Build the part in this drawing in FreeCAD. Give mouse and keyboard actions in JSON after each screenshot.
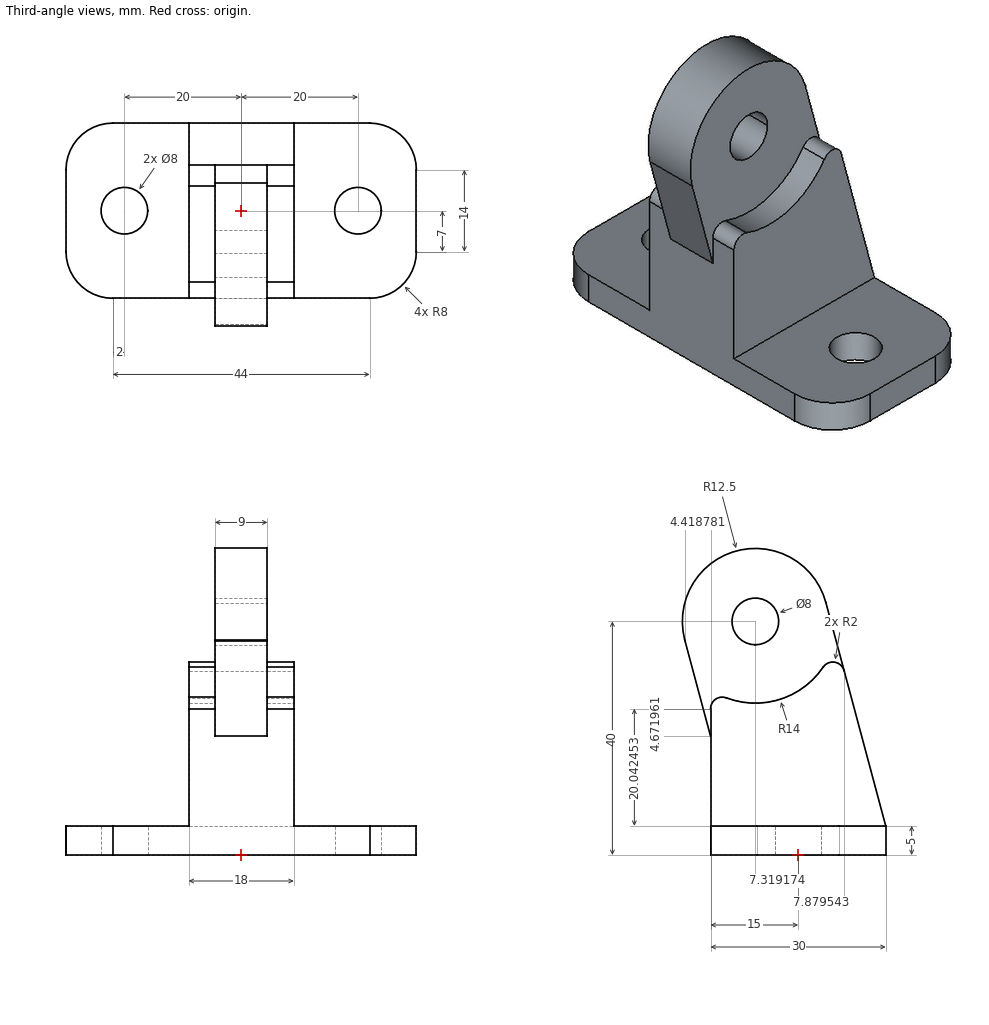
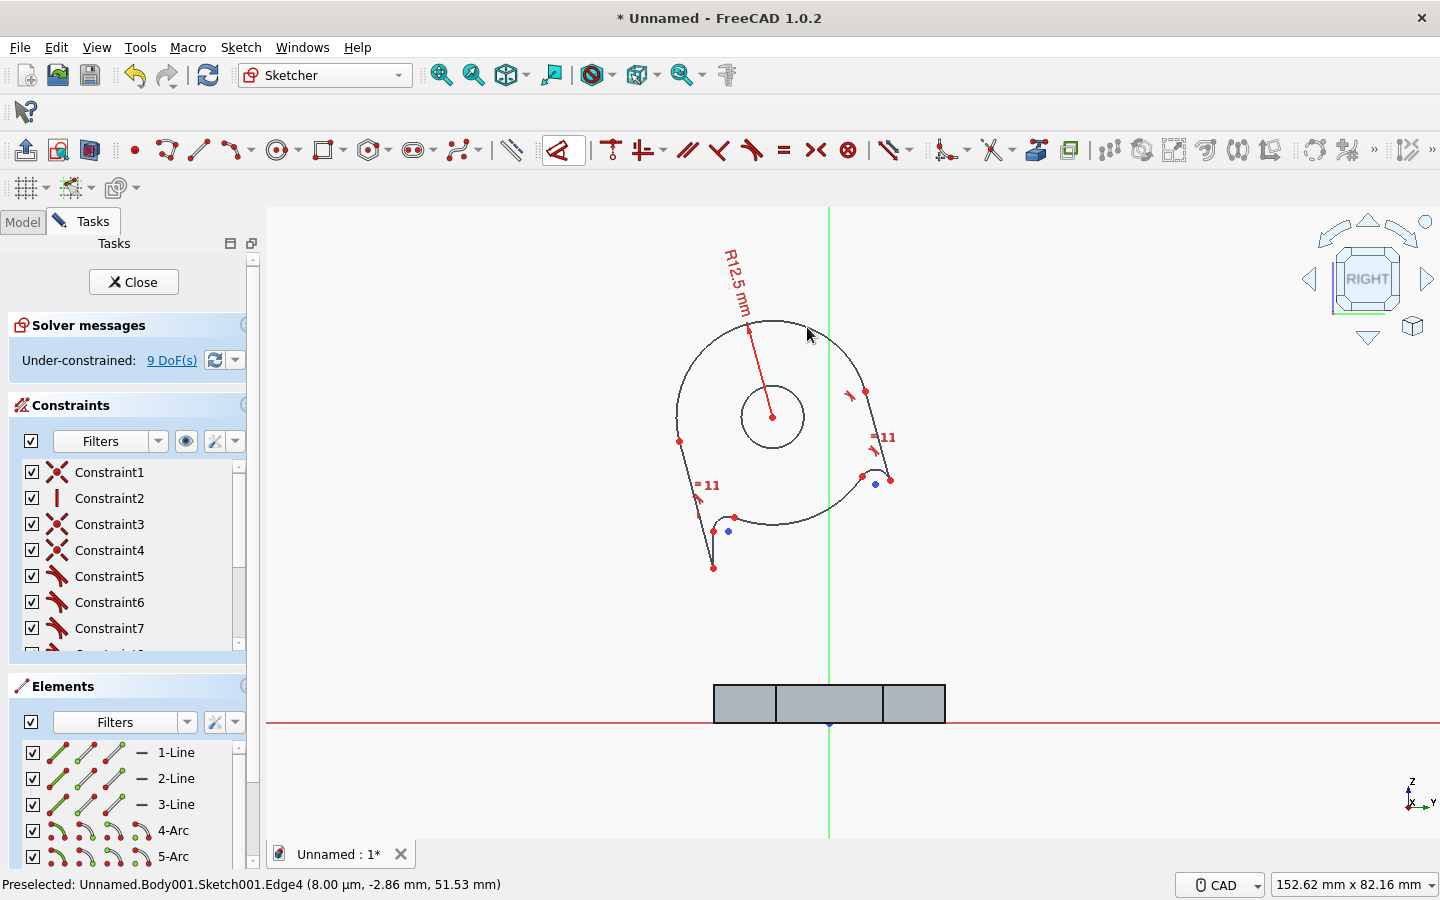
{"action": "scroll", "coordinate": [720, 519], "scroll_direction": "up", "scroll_amount": 5}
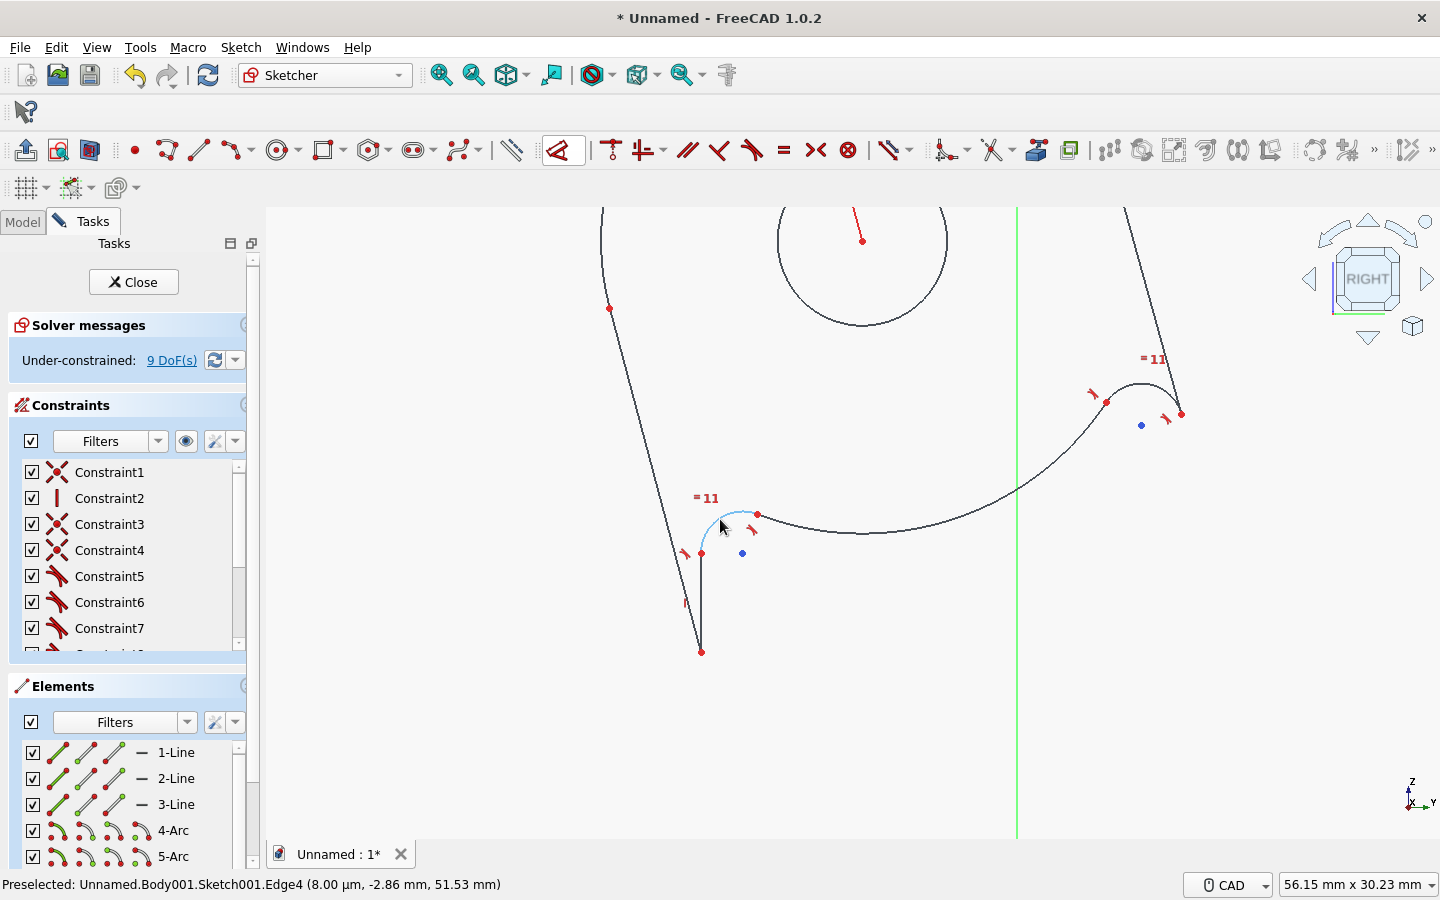
{"action": "left_click", "coordinate": [719, 519]}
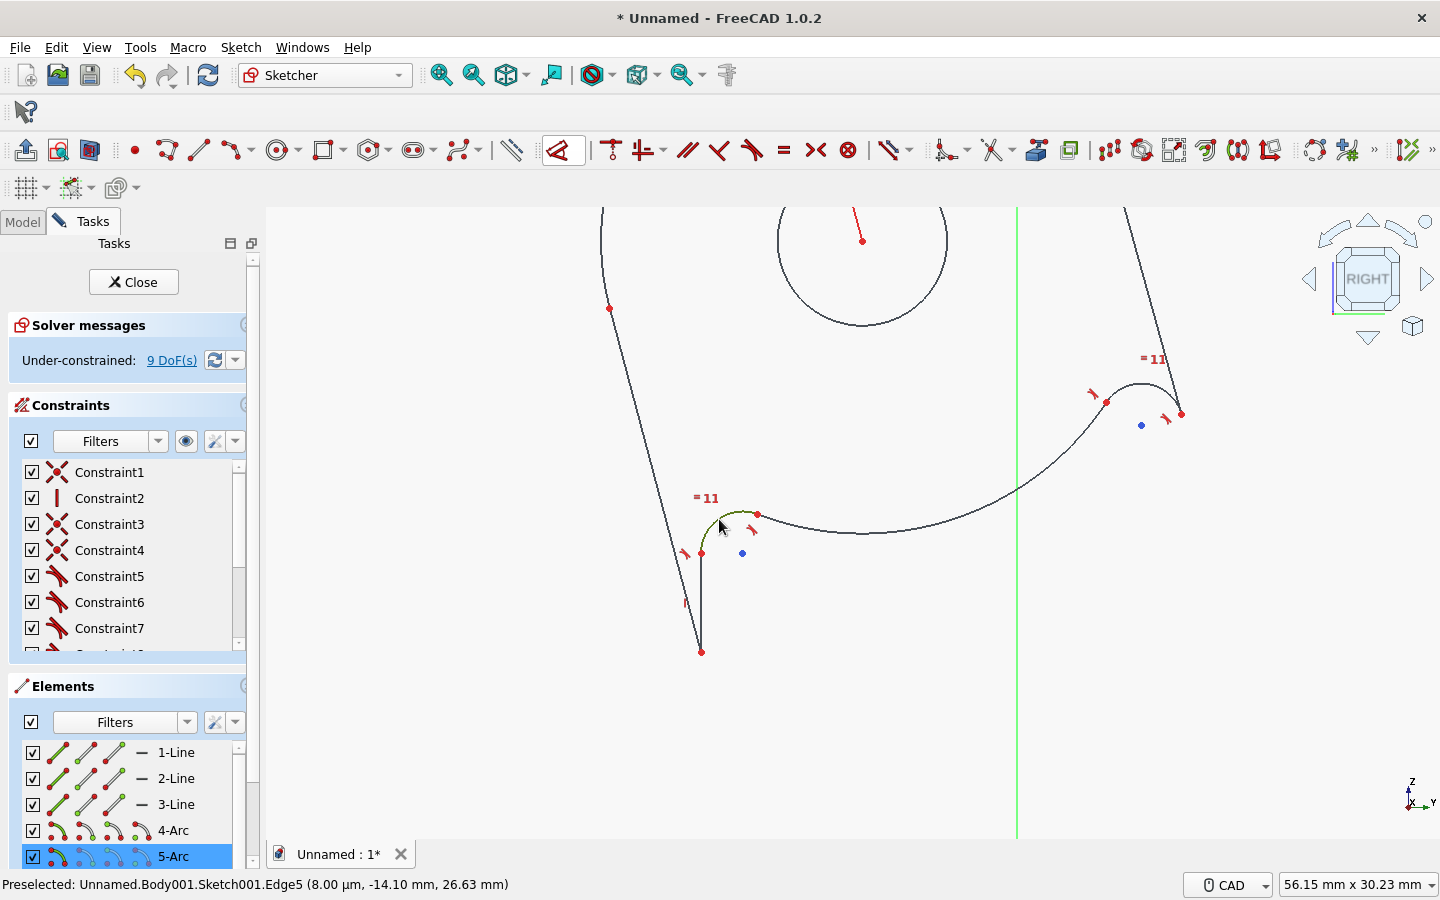
{"action": "key", "text": "k r"}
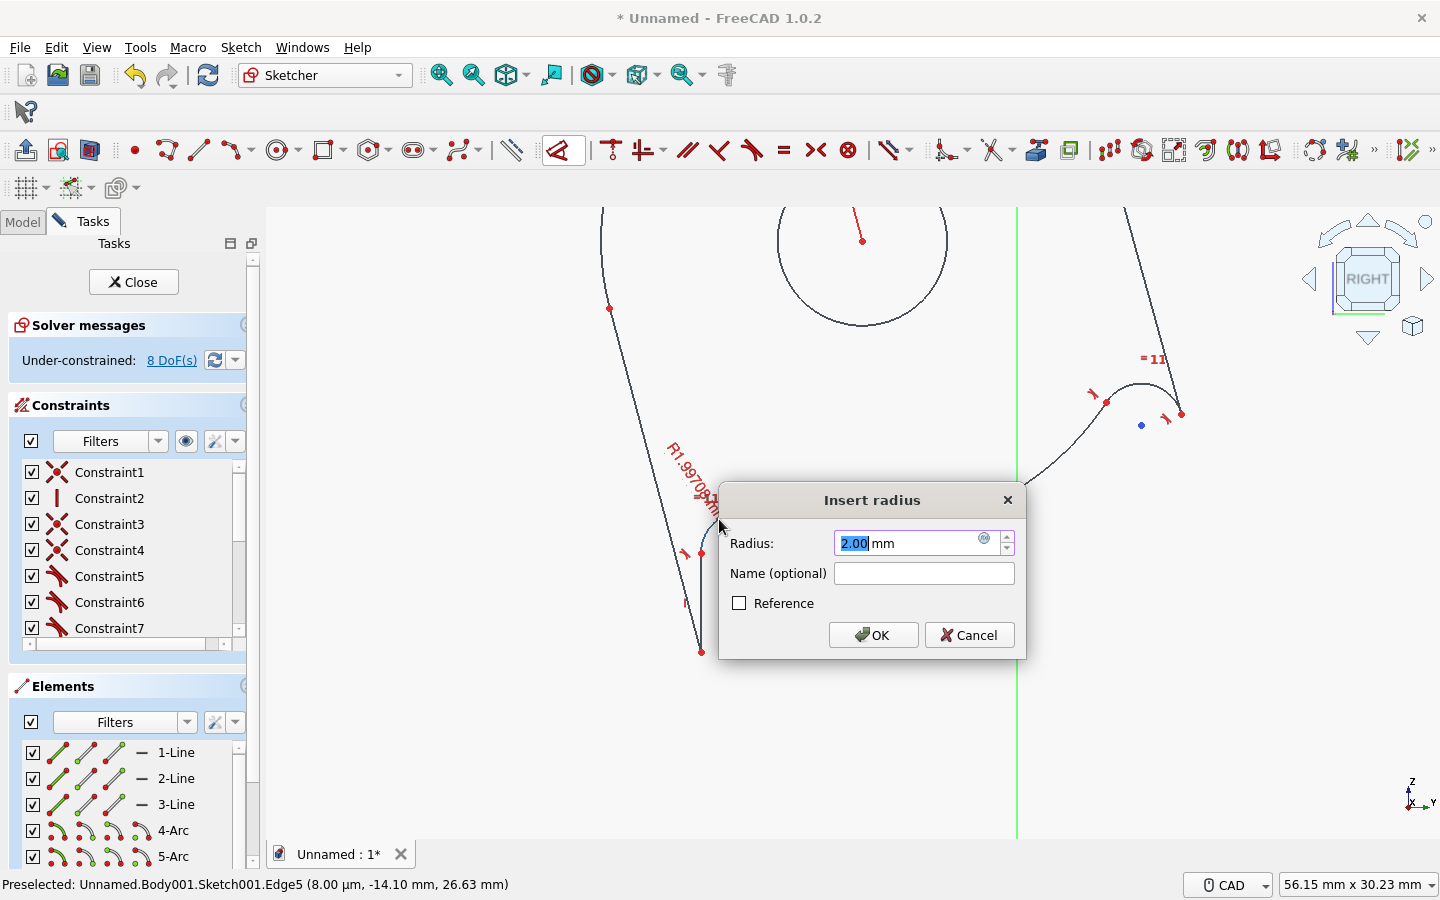
{"action": "type", "text": "2"}
{"action": "key", "text": "Return"}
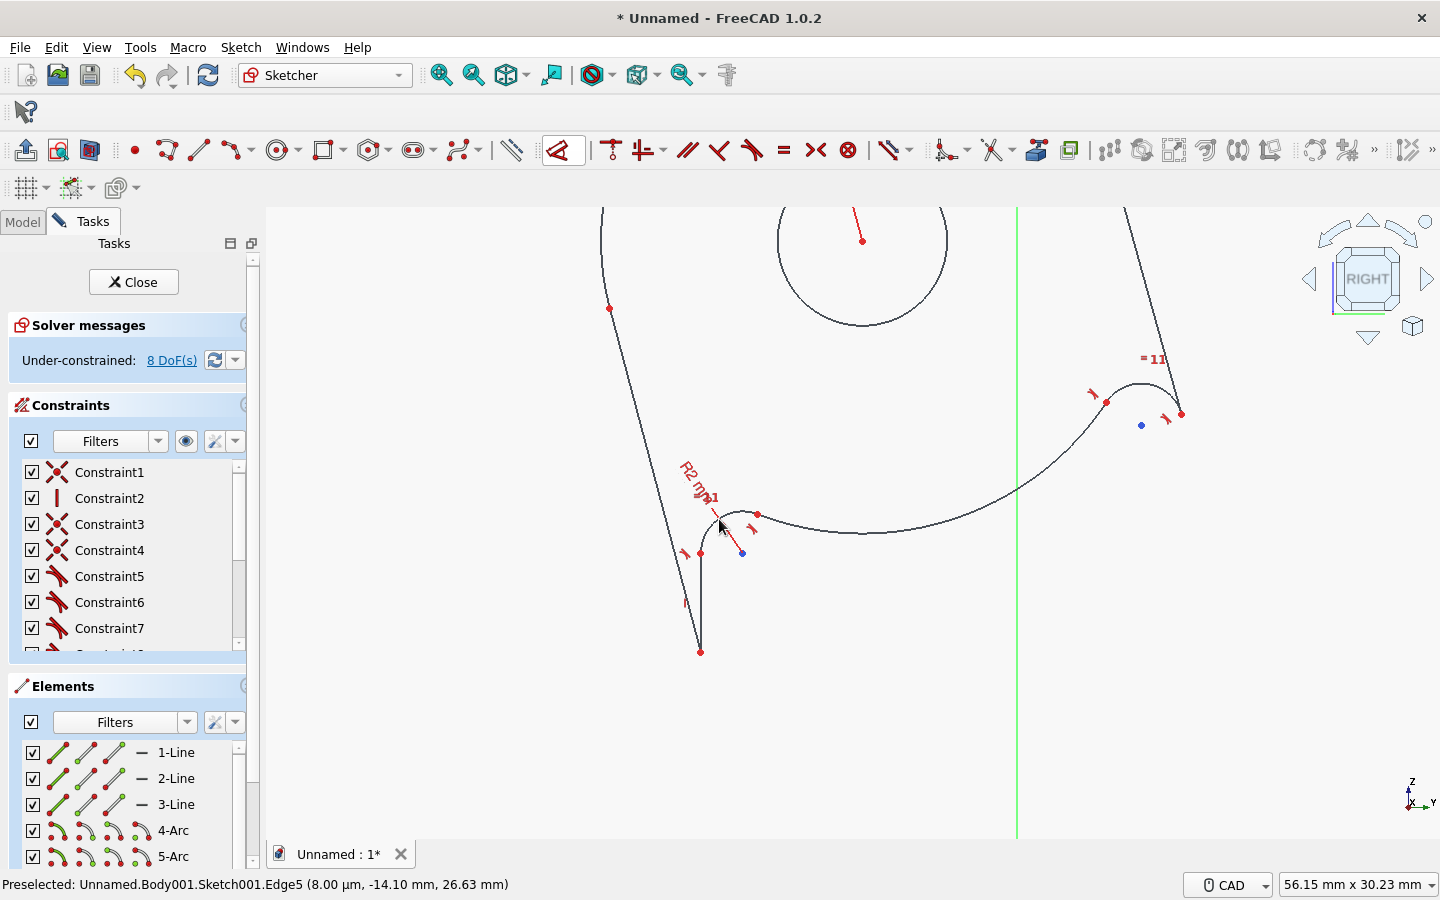
{"action": "left_click", "coordinate": [874, 533]}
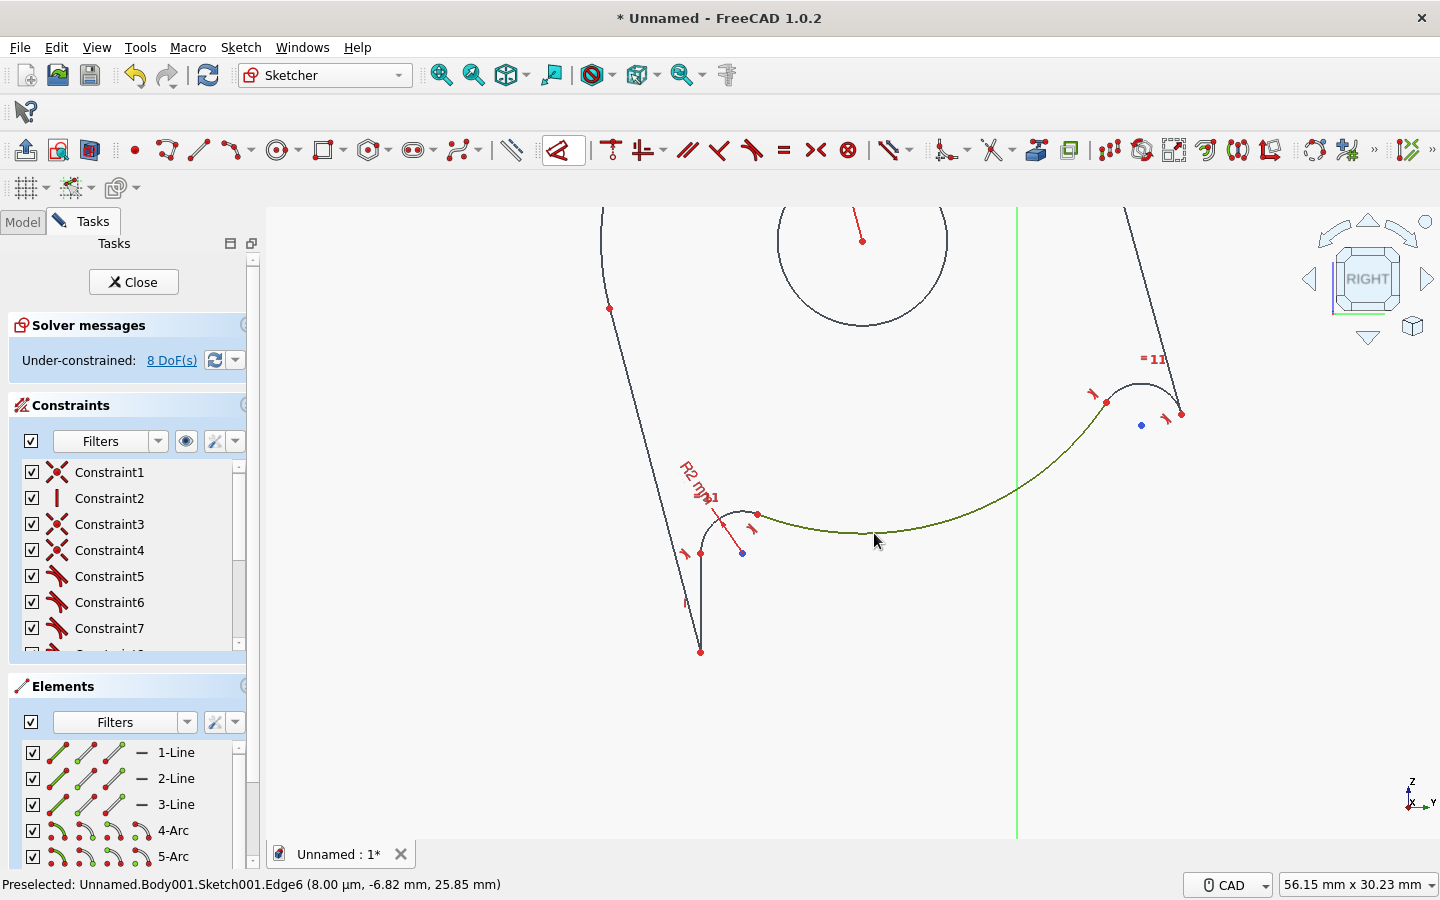
{"action": "key", "text": "k r"}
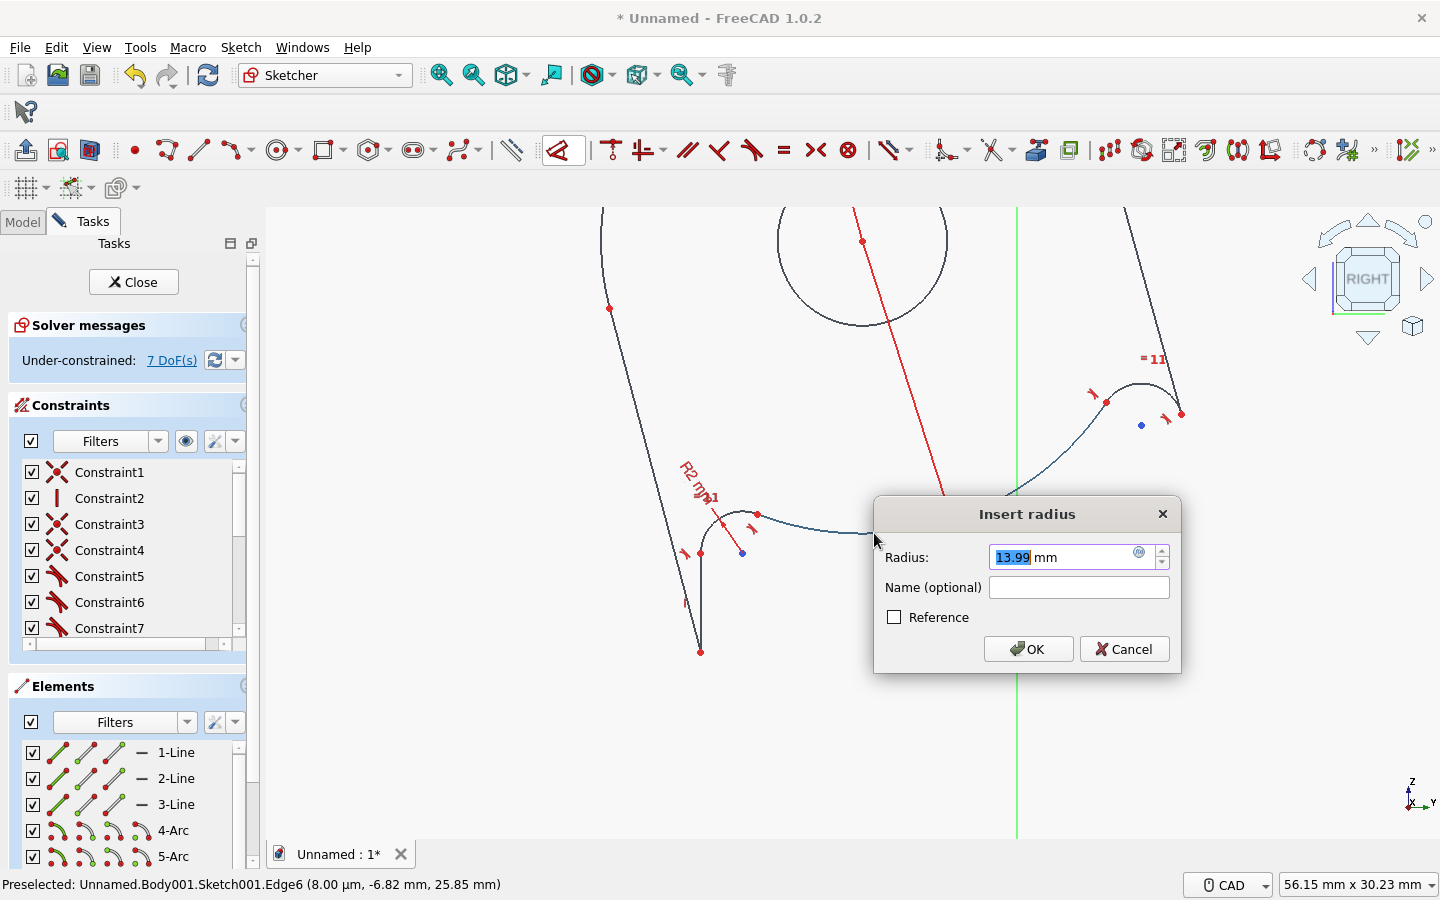
{"action": "type", "text": "14"}
{"action": "key", "text": "Return"}